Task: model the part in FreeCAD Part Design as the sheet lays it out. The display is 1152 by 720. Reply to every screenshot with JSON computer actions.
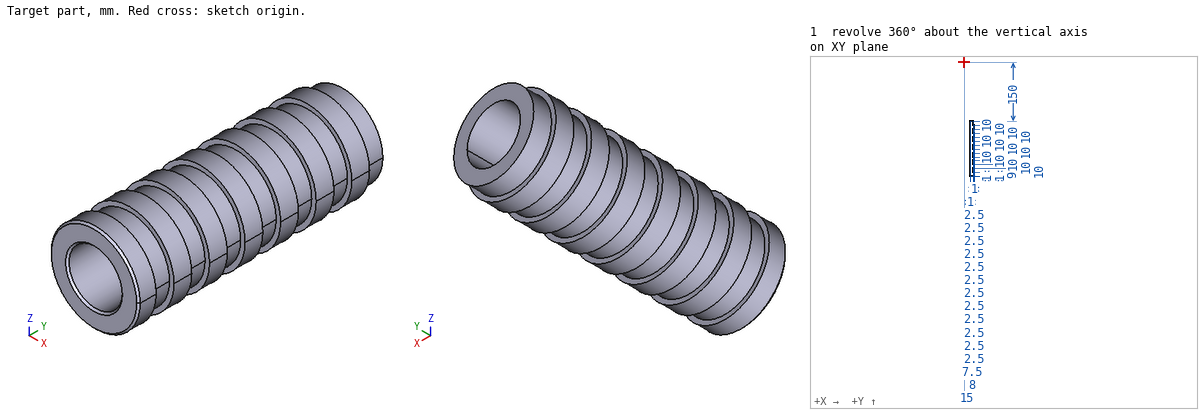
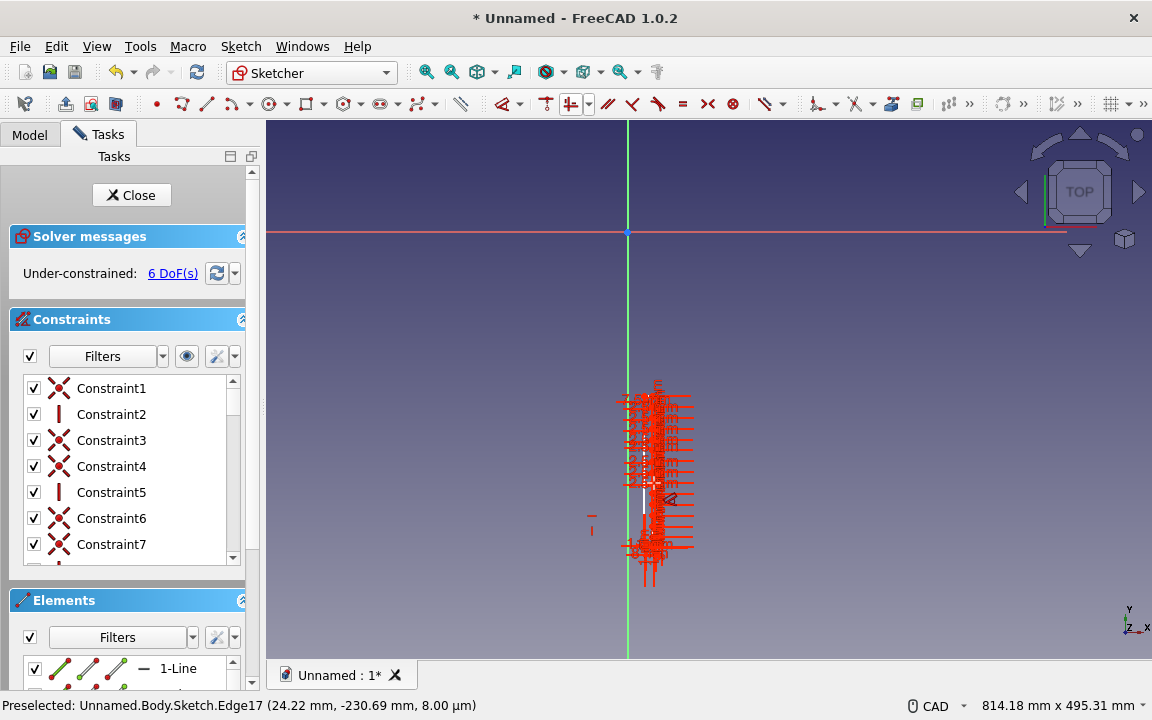
{"action": "scroll", "coordinate": [653, 494], "scroll_direction": "up", "scroll_amount": 14}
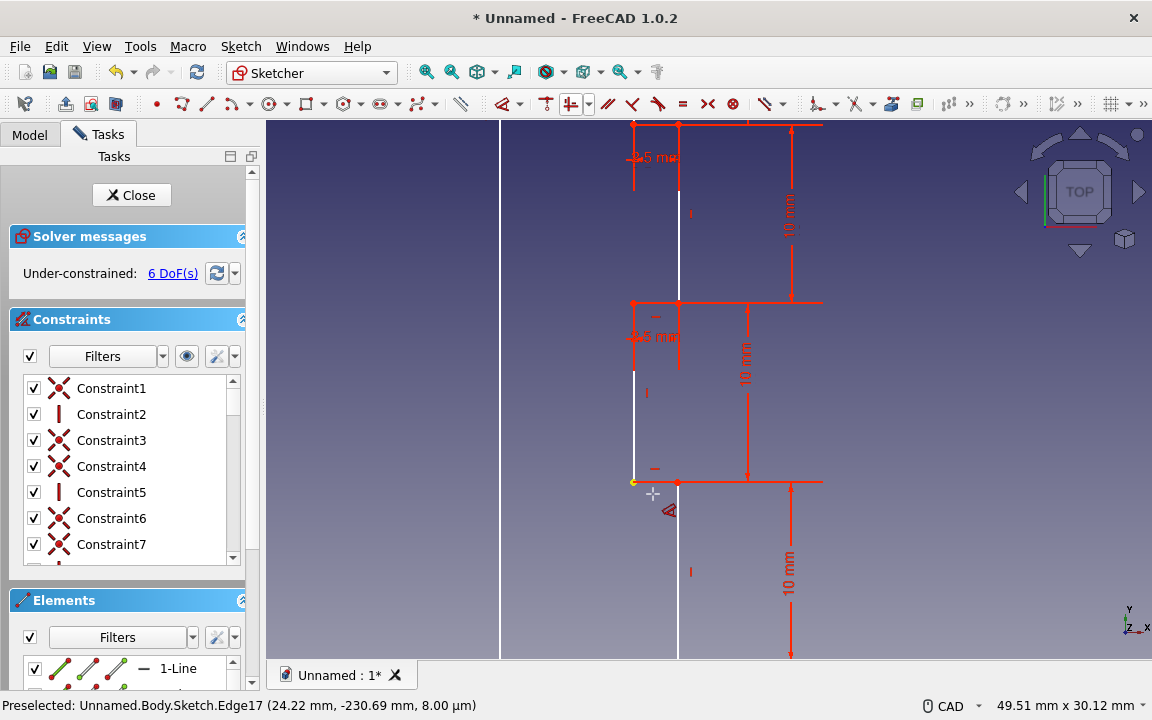
{"action": "left_click", "coordinate": [647, 482]}
{"action": "left_click", "coordinate": [656, 516]}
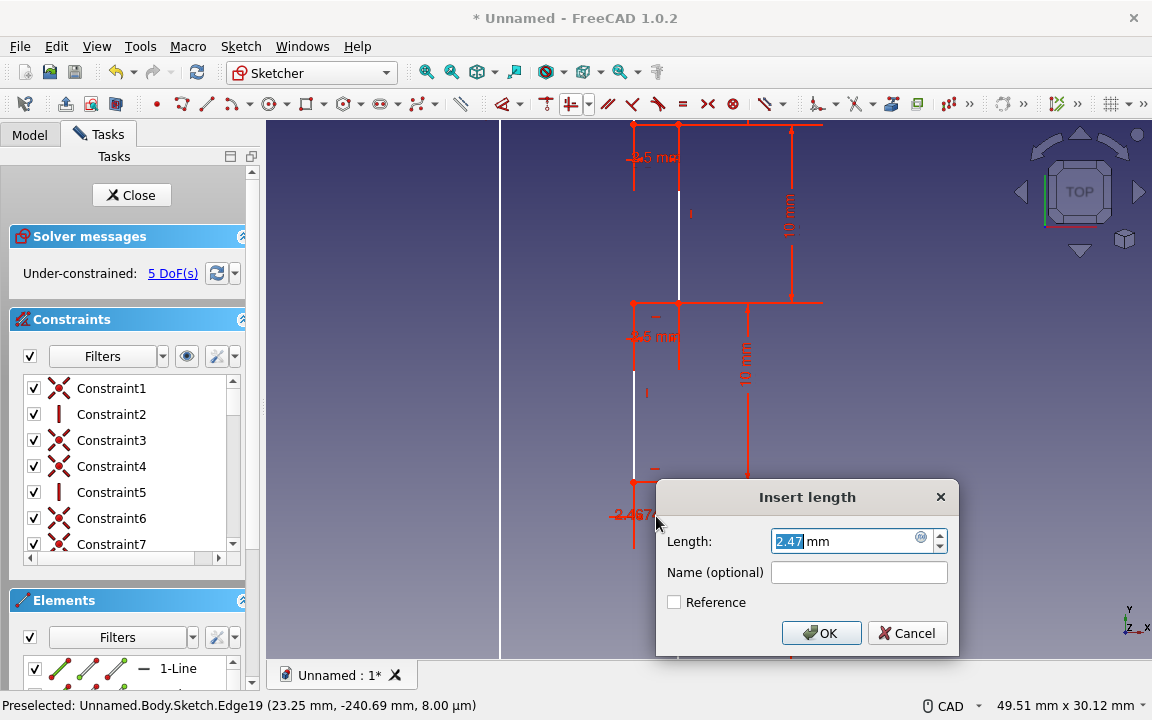
{"action": "type", "text": "2.5"}
{"action": "key", "text": "Return"}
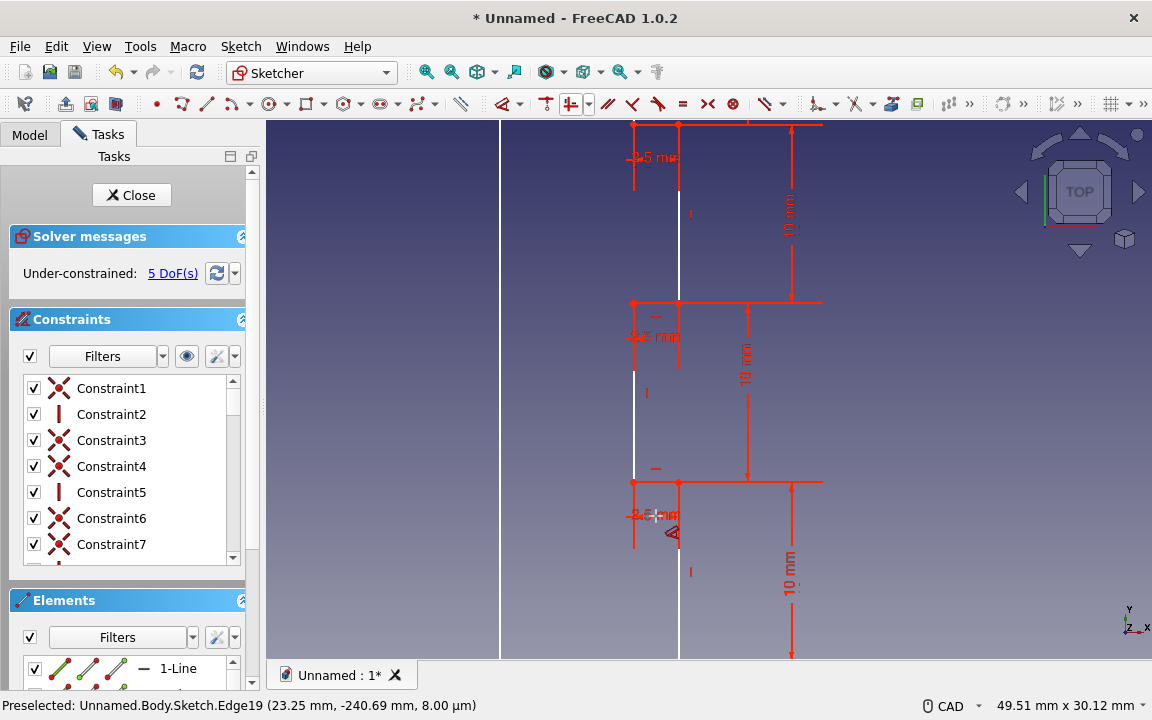
{"action": "scroll", "coordinate": [653, 494], "scroll_direction": "down", "scroll_amount": 14}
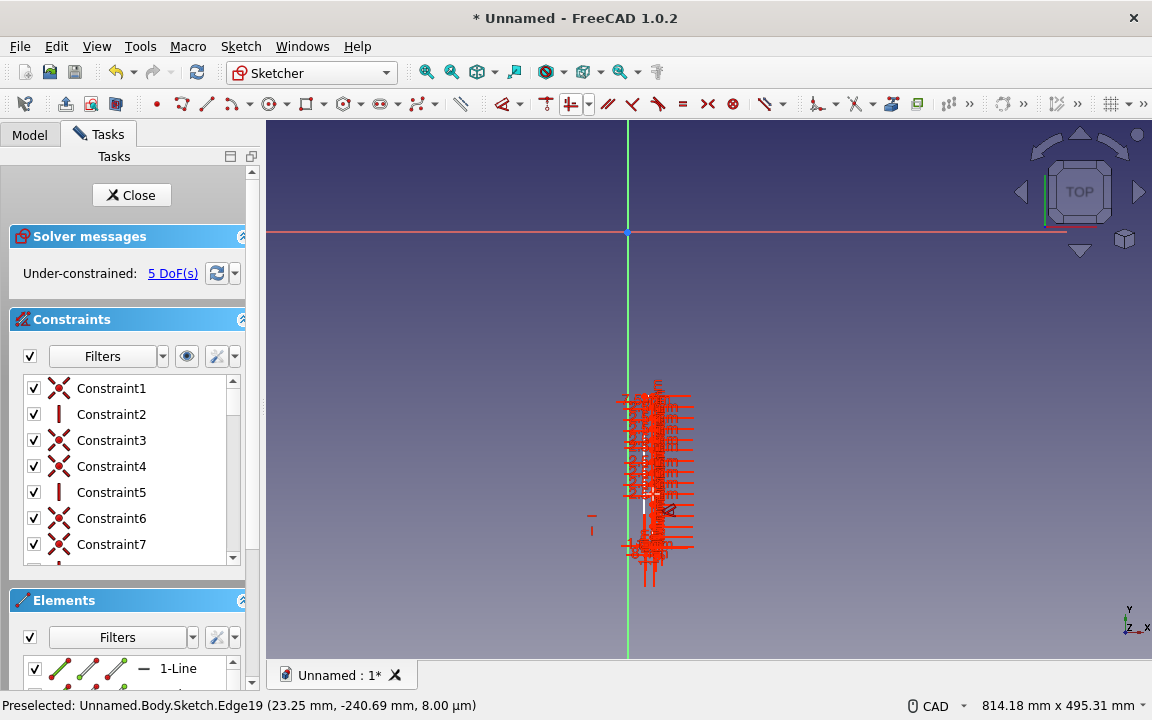
{"action": "scroll", "coordinate": [654, 505], "scroll_direction": "up", "scroll_amount": 14}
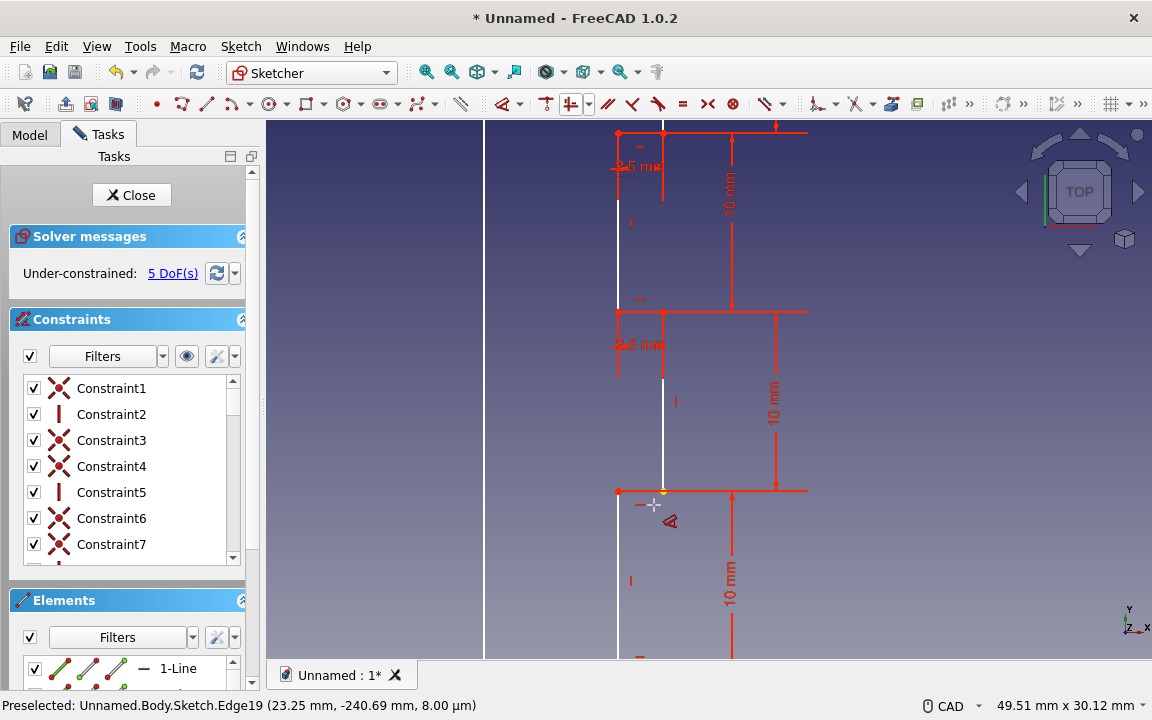
{"action": "left_click", "coordinate": [650, 491]}
{"action": "left_click", "coordinate": [641, 525]}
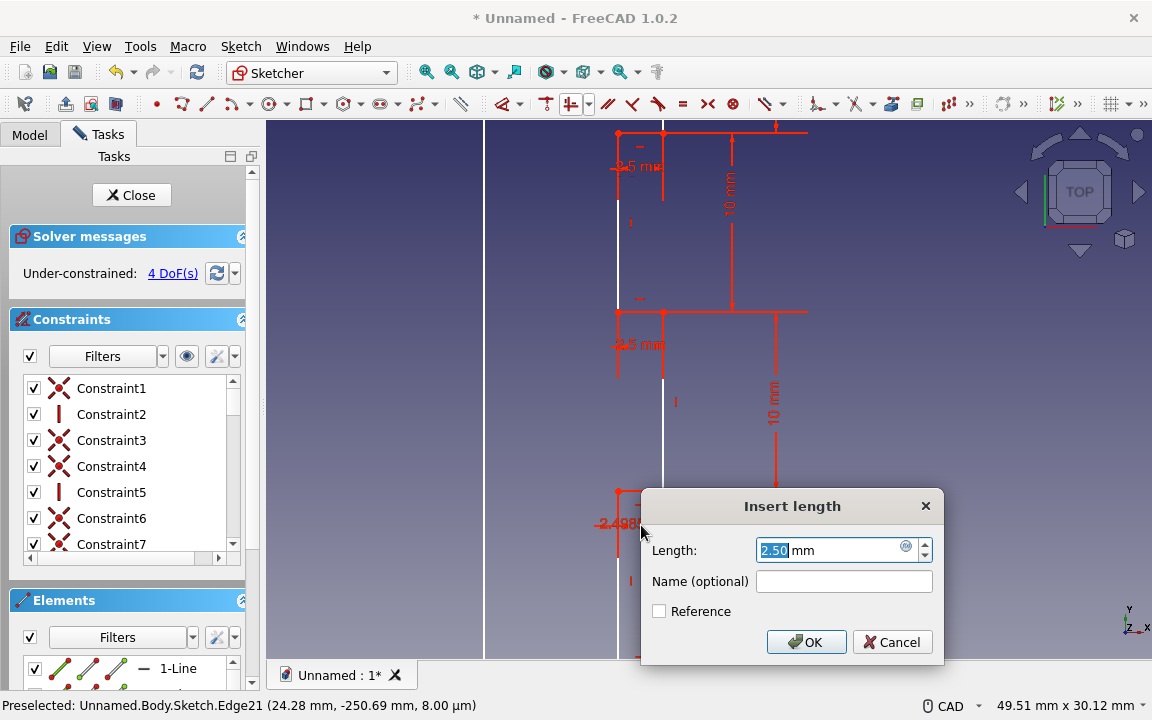
{"action": "type", "text": "2.5"}
{"action": "key", "text": "Return"}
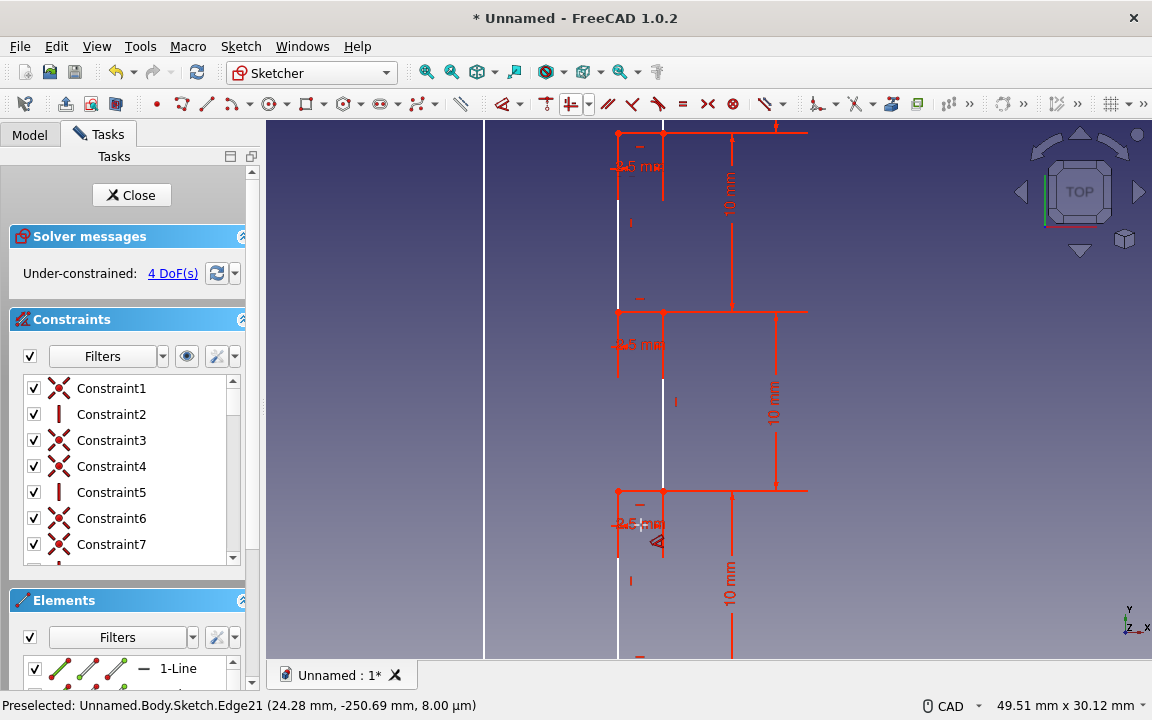
{"action": "scroll", "coordinate": [654, 505], "scroll_direction": "down", "scroll_amount": 14}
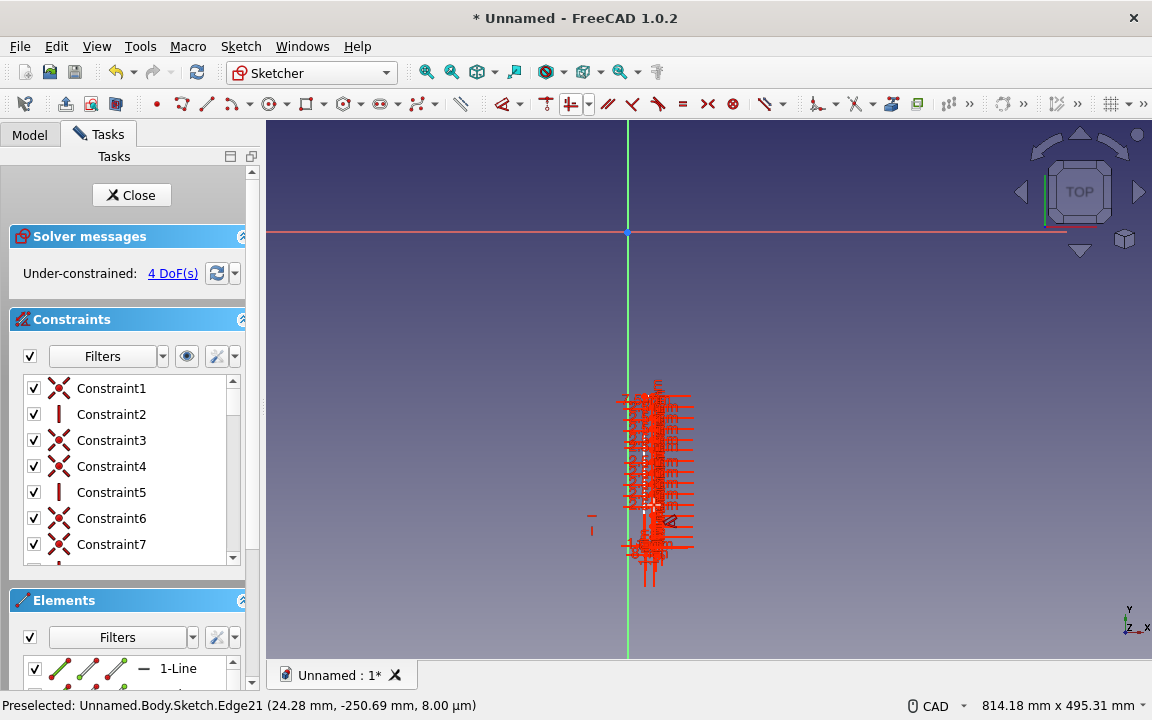
{"action": "scroll", "coordinate": [653, 516], "scroll_direction": "up", "scroll_amount": 14}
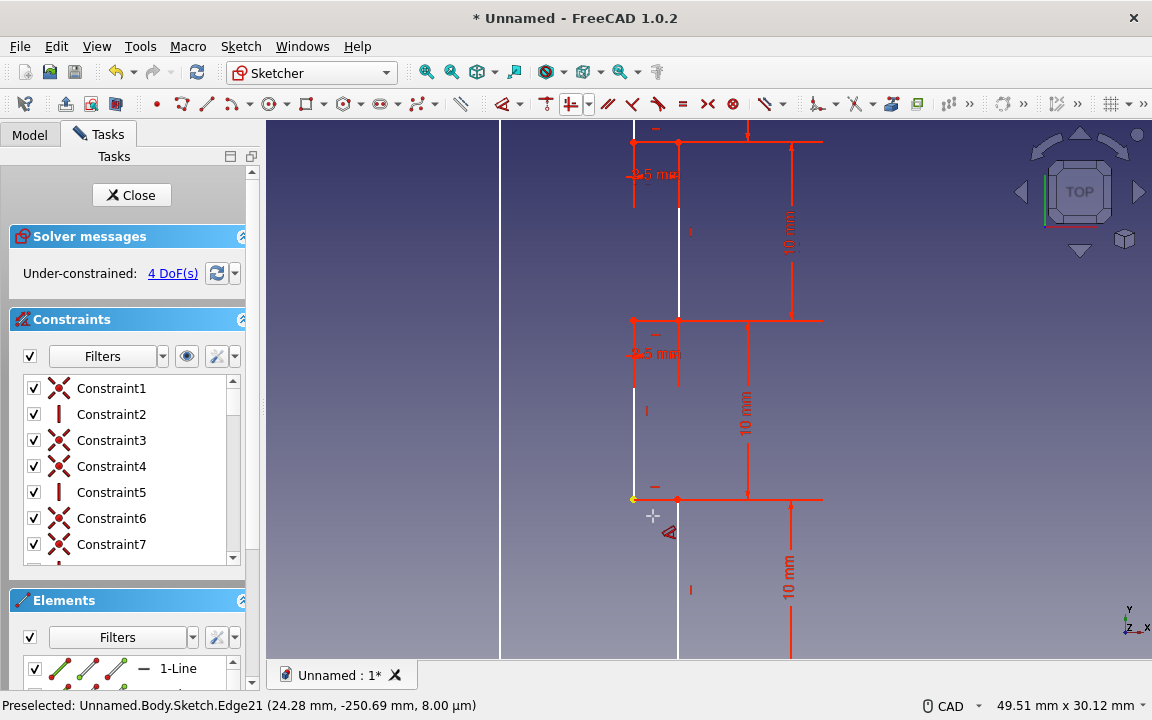
{"action": "left_click", "coordinate": [647, 500]}
{"action": "left_click", "coordinate": [656, 534]}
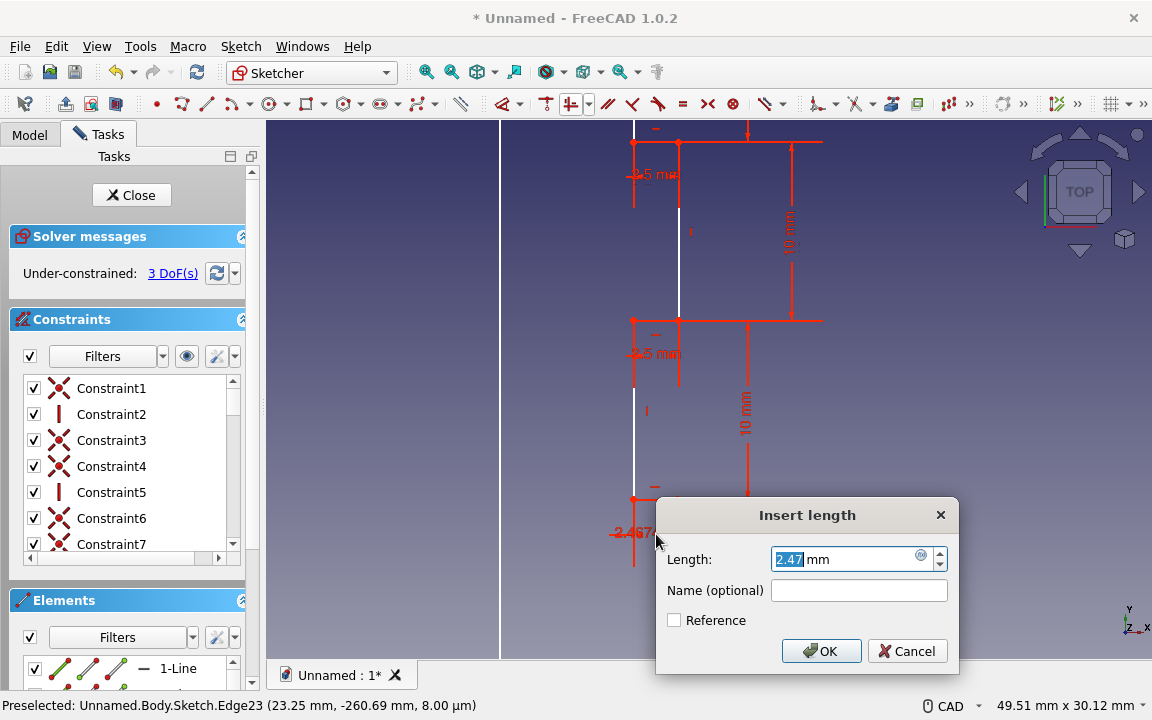
{"action": "type", "text": "2.5"}
{"action": "key", "text": "Return"}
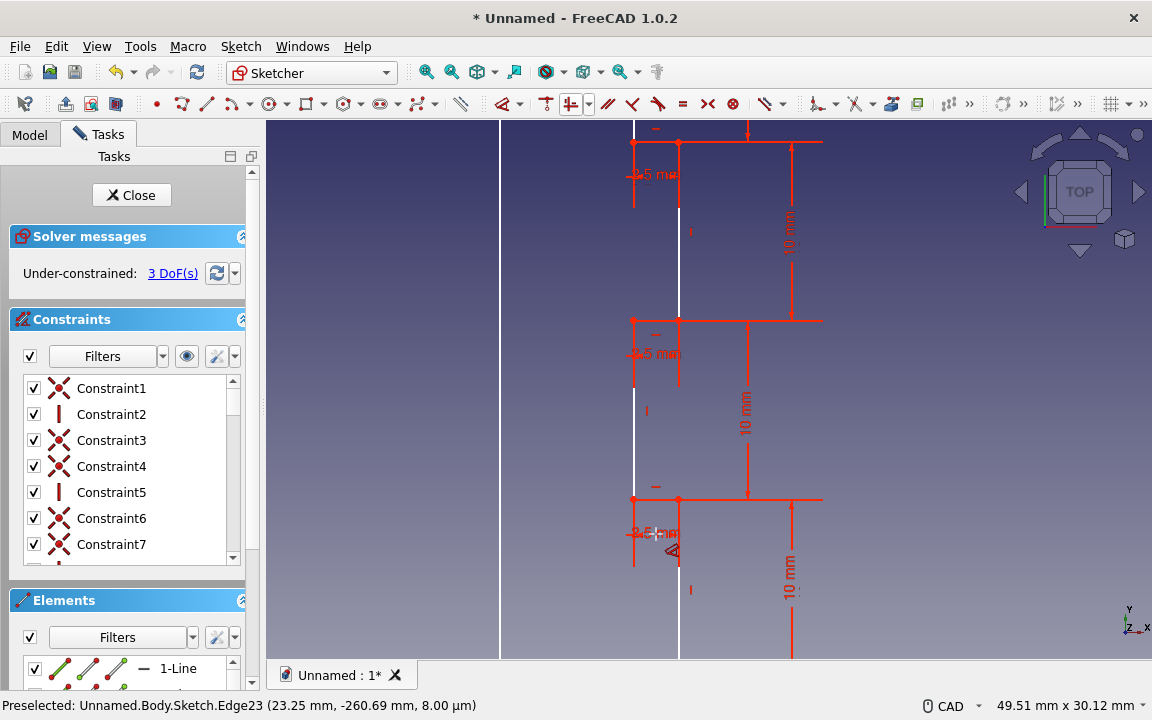
{"action": "scroll", "coordinate": [653, 516], "scroll_direction": "down", "scroll_amount": 14}